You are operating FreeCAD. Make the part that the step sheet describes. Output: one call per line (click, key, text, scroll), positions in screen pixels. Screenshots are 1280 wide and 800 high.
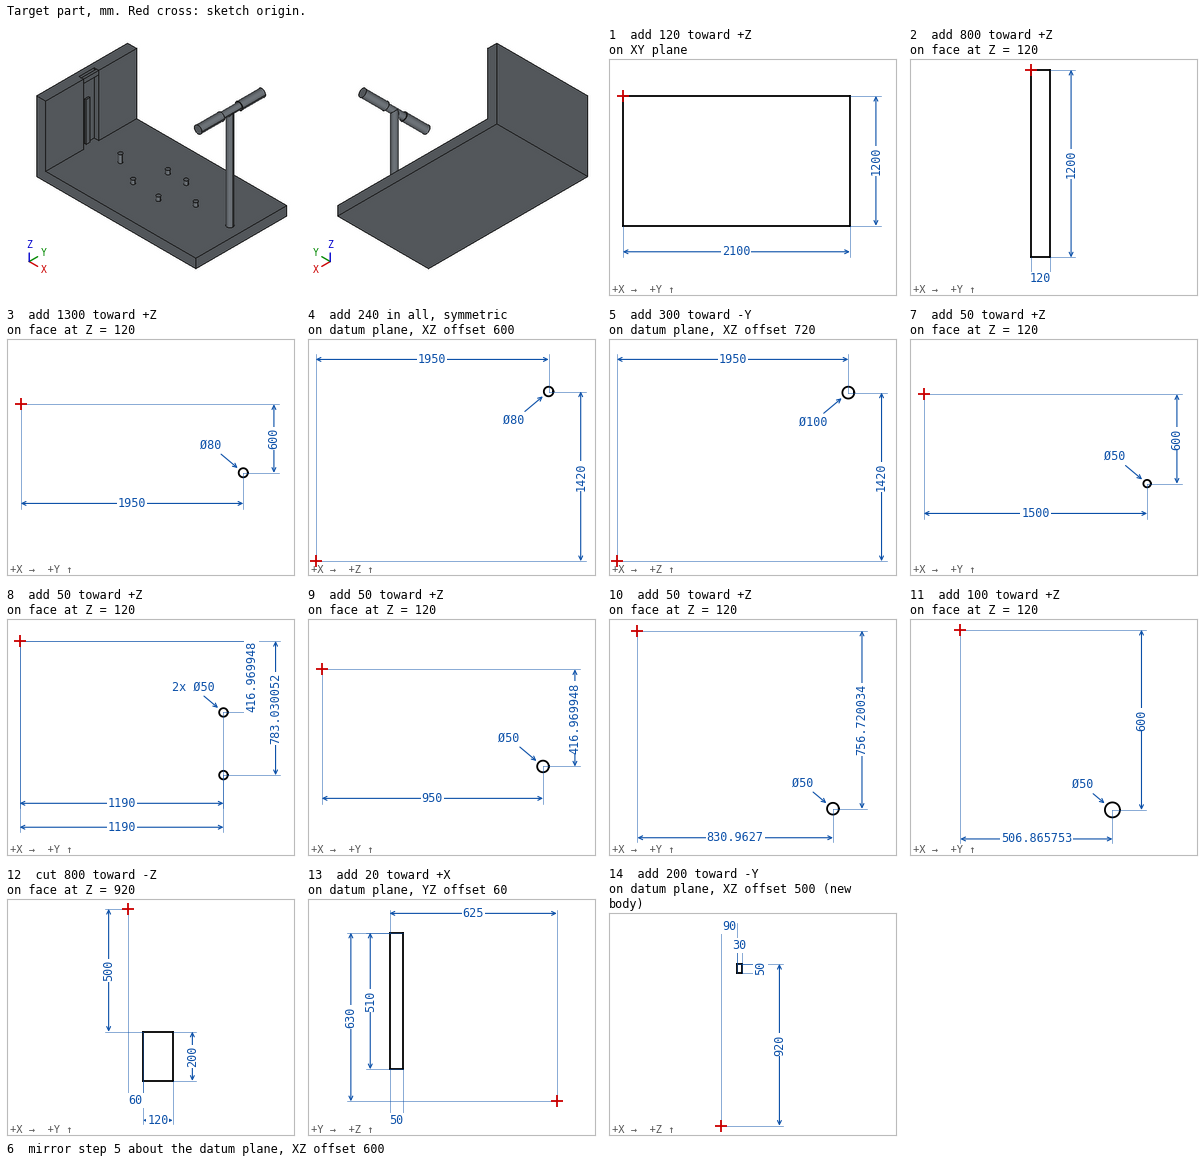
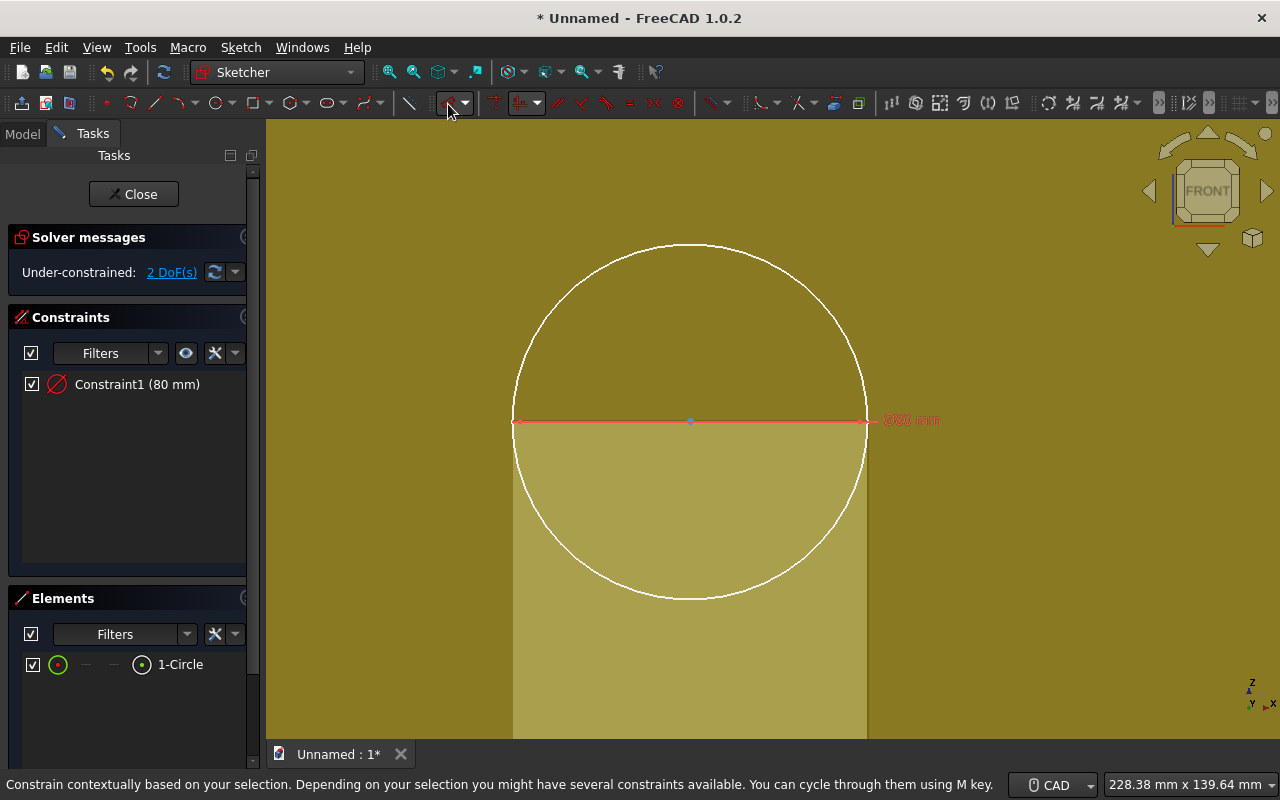
click(690, 422)
click(492, 388)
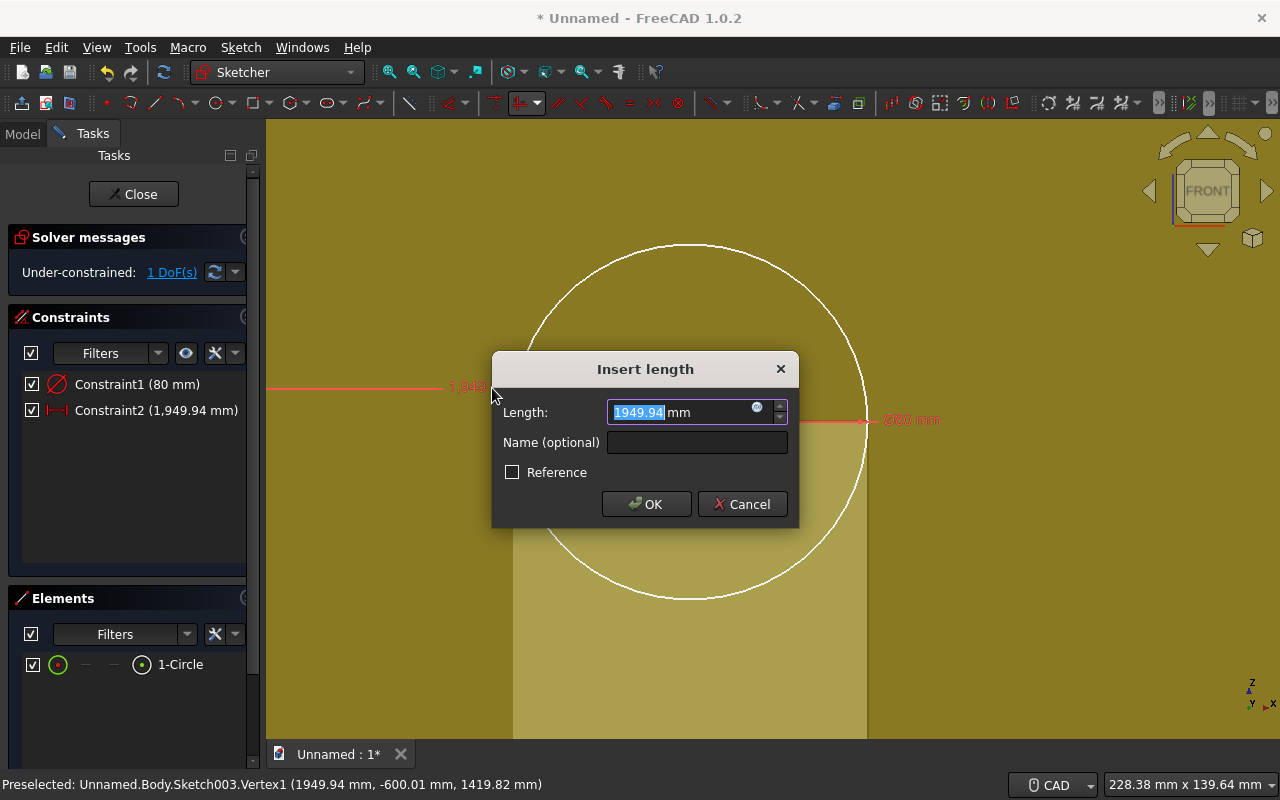
text(1950)
key(Return)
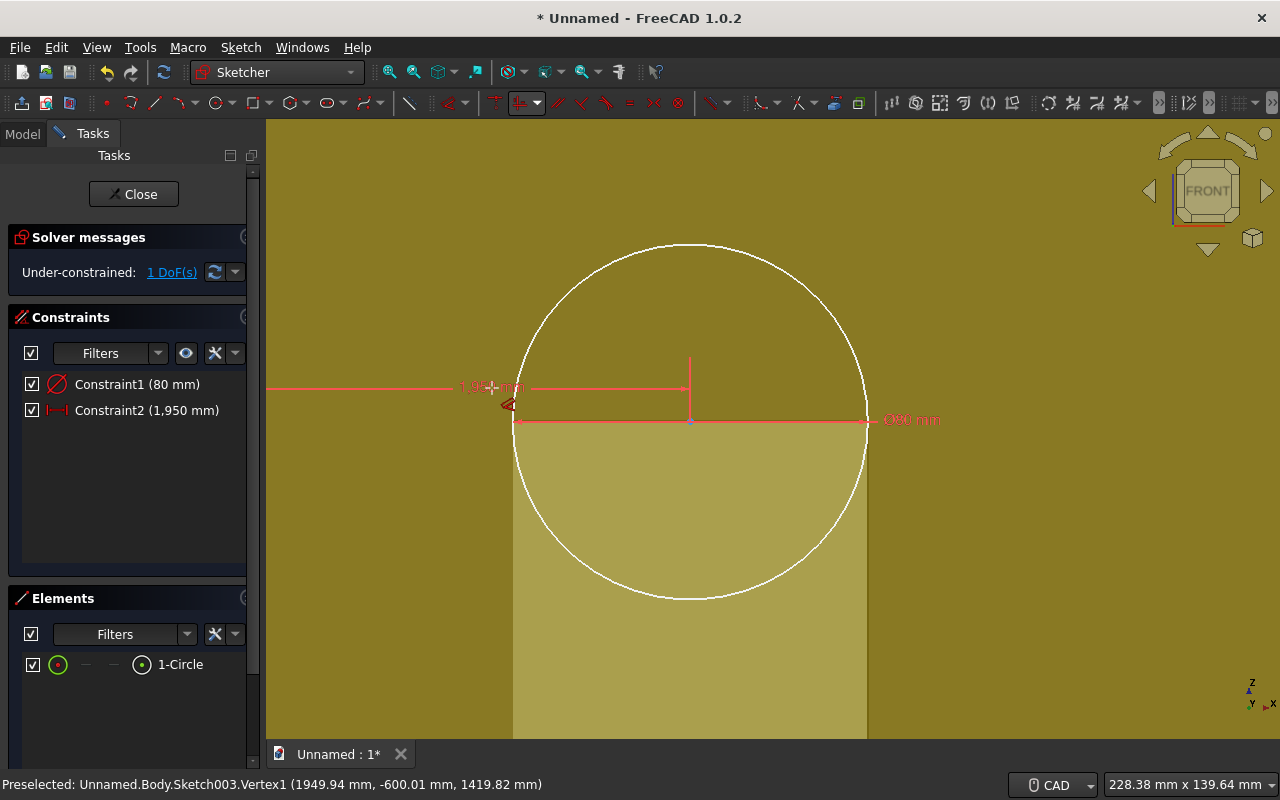
click(690, 422)
click(724, 567)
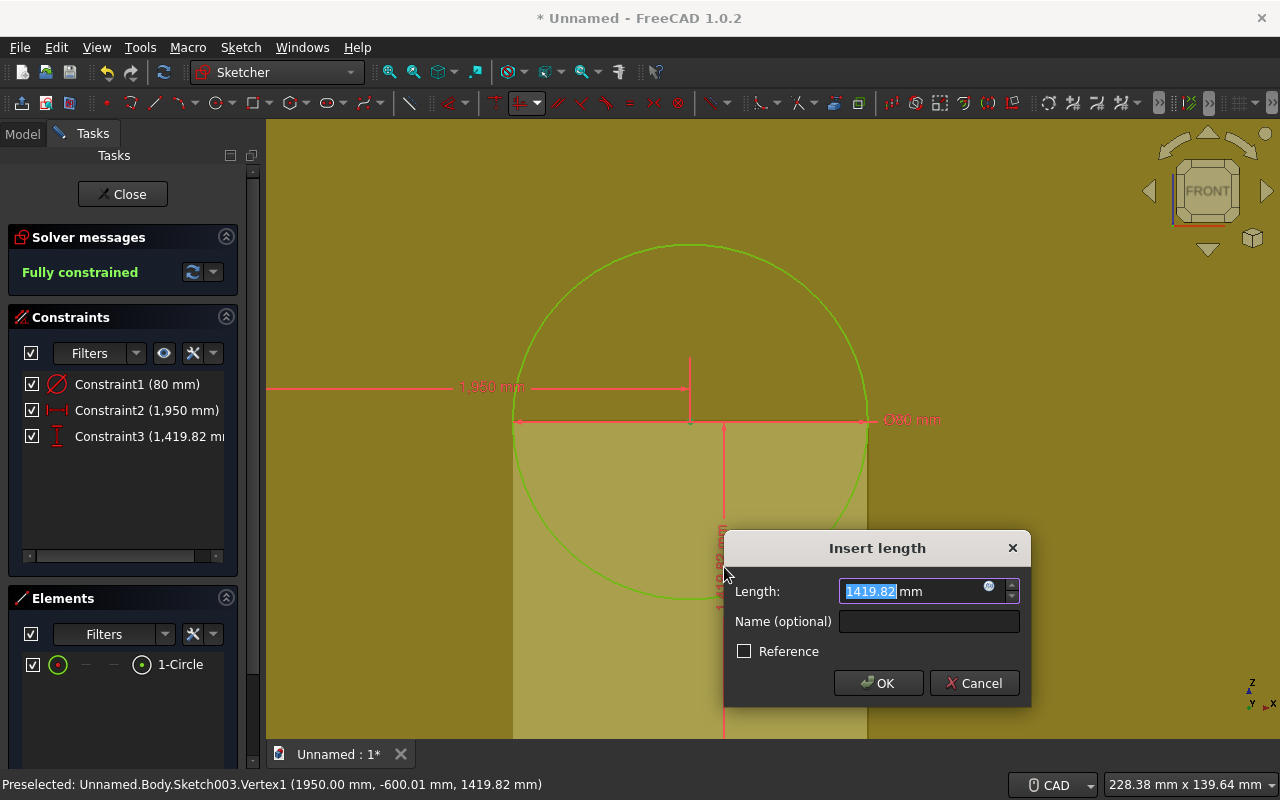
text(1420)
key(Return)
key(Escape)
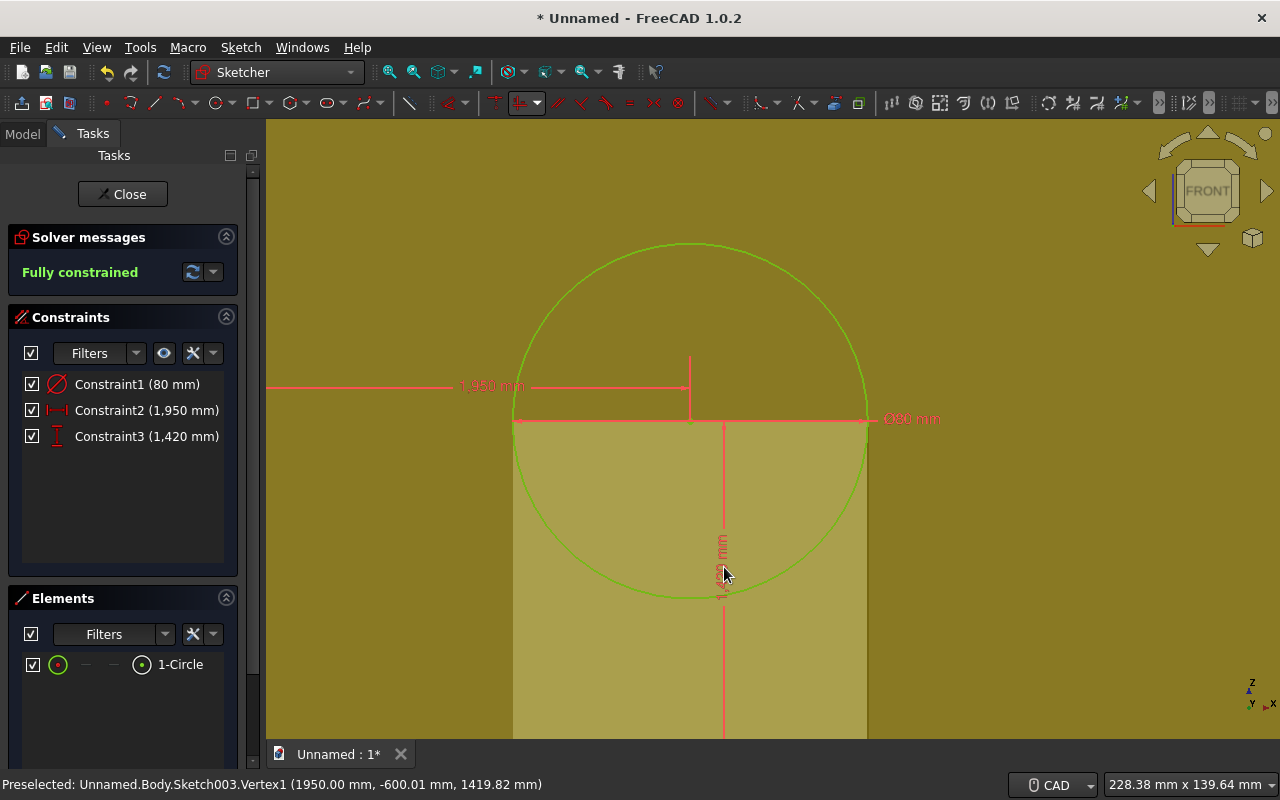
click(123, 194)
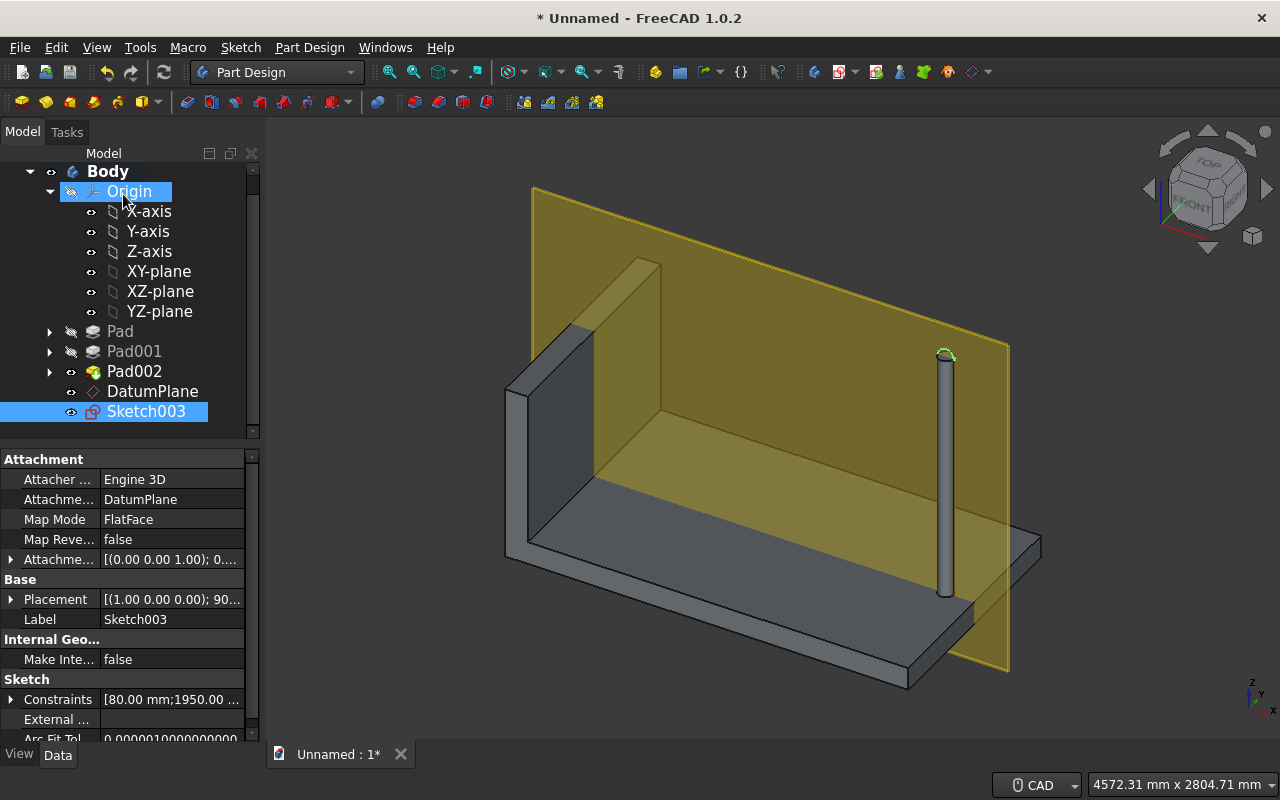
click(22, 102)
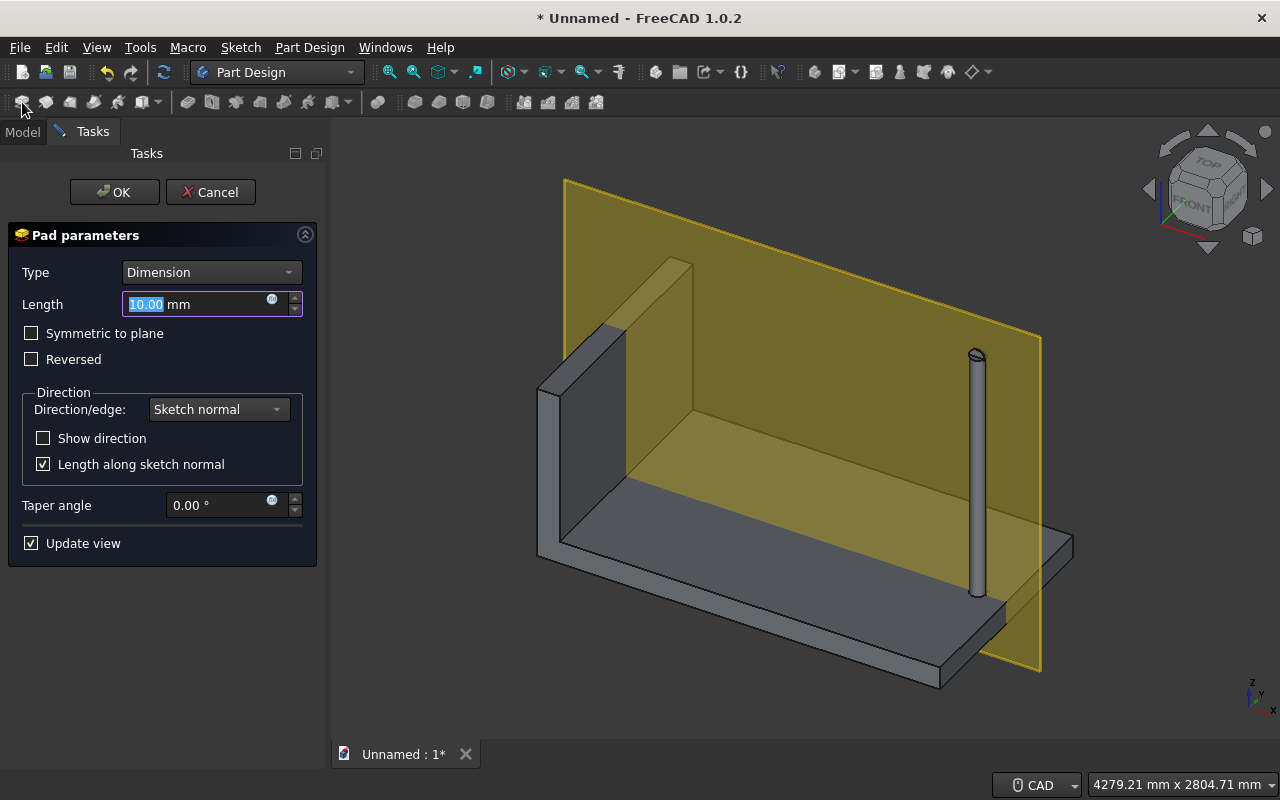
text(240)
key(Tab)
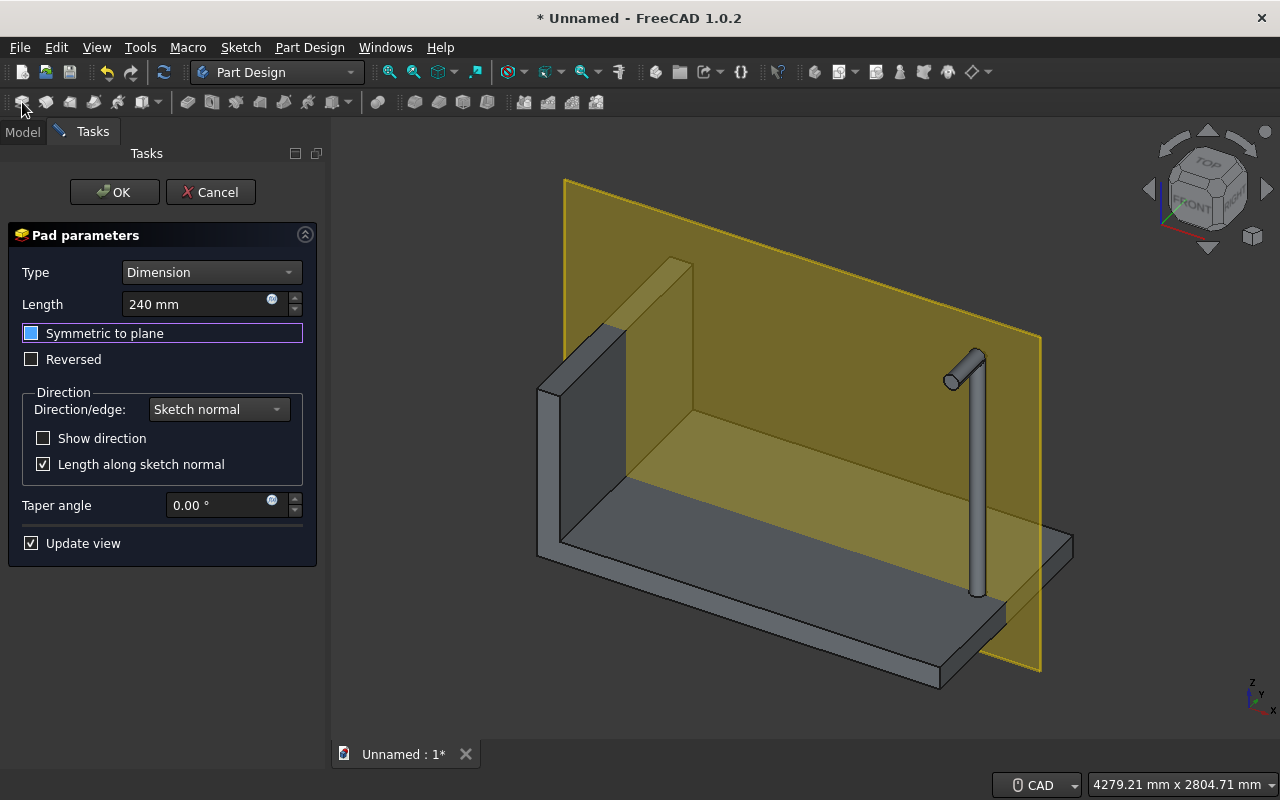
click(30, 333)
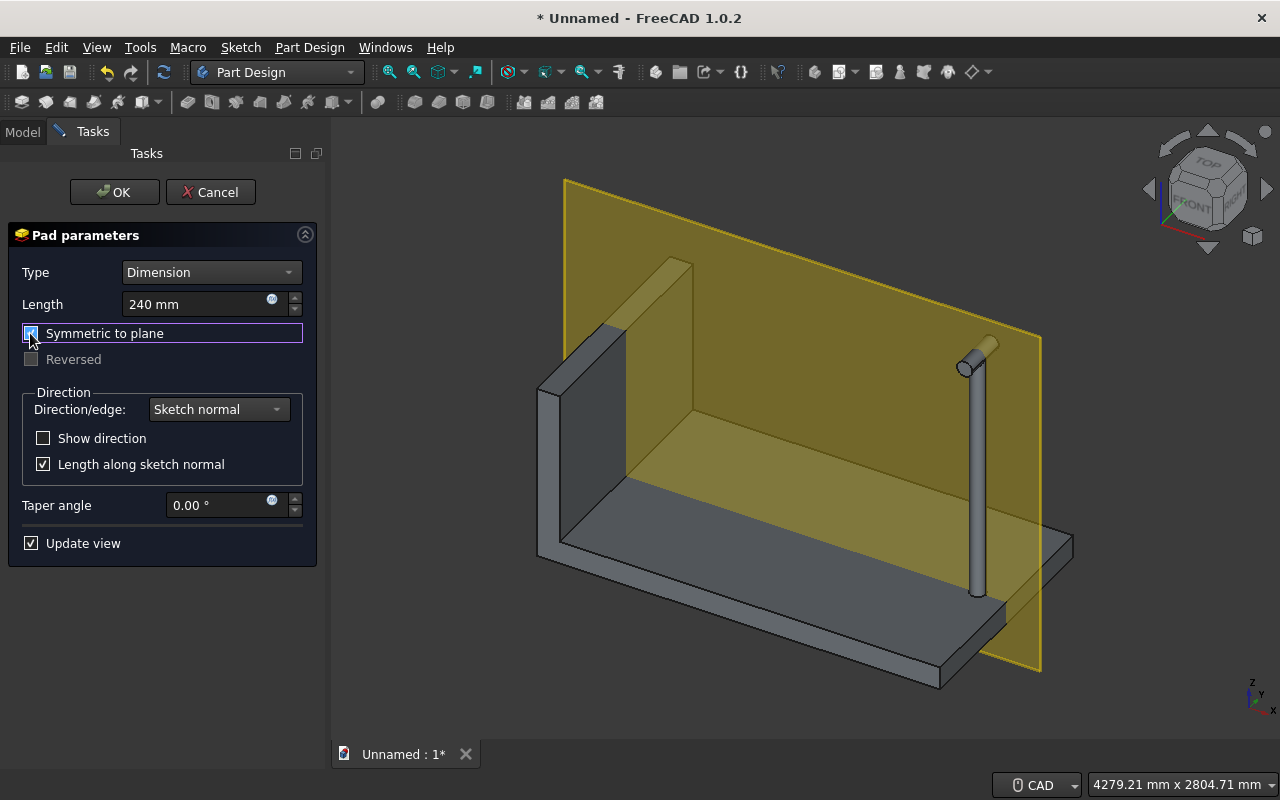
click(115, 192)